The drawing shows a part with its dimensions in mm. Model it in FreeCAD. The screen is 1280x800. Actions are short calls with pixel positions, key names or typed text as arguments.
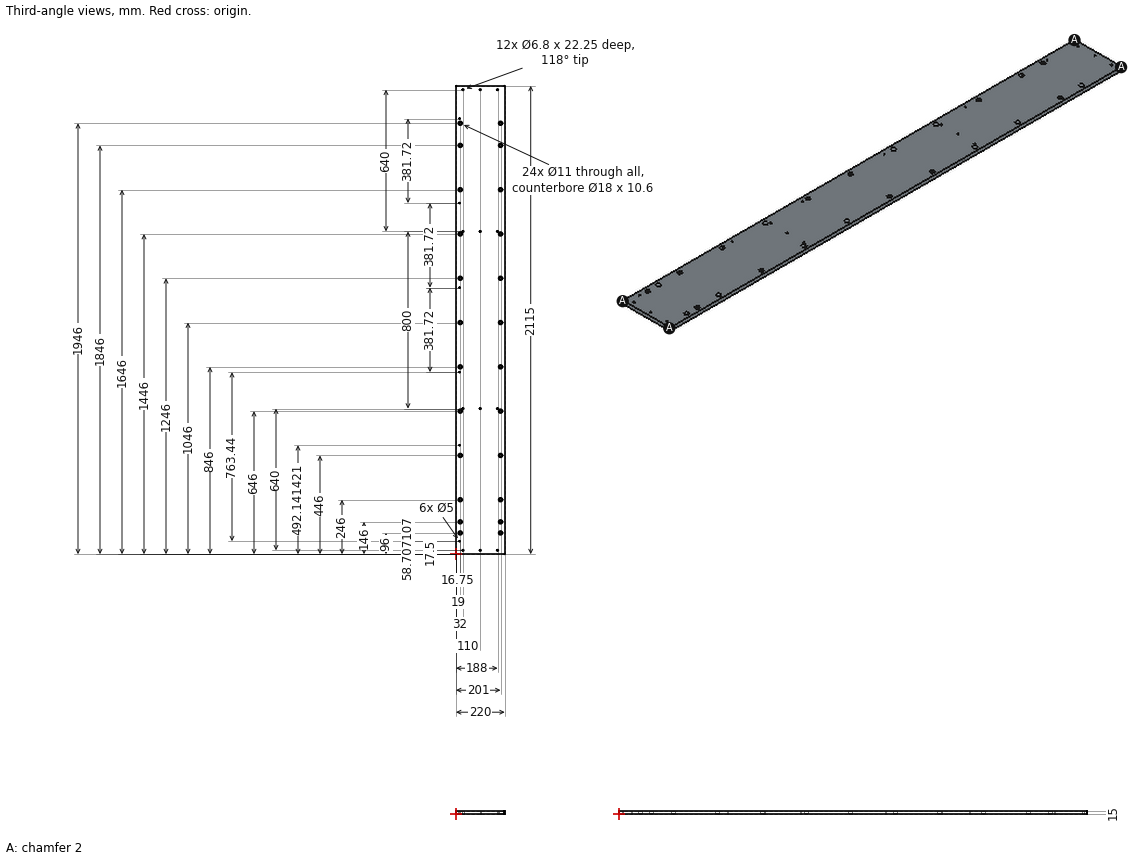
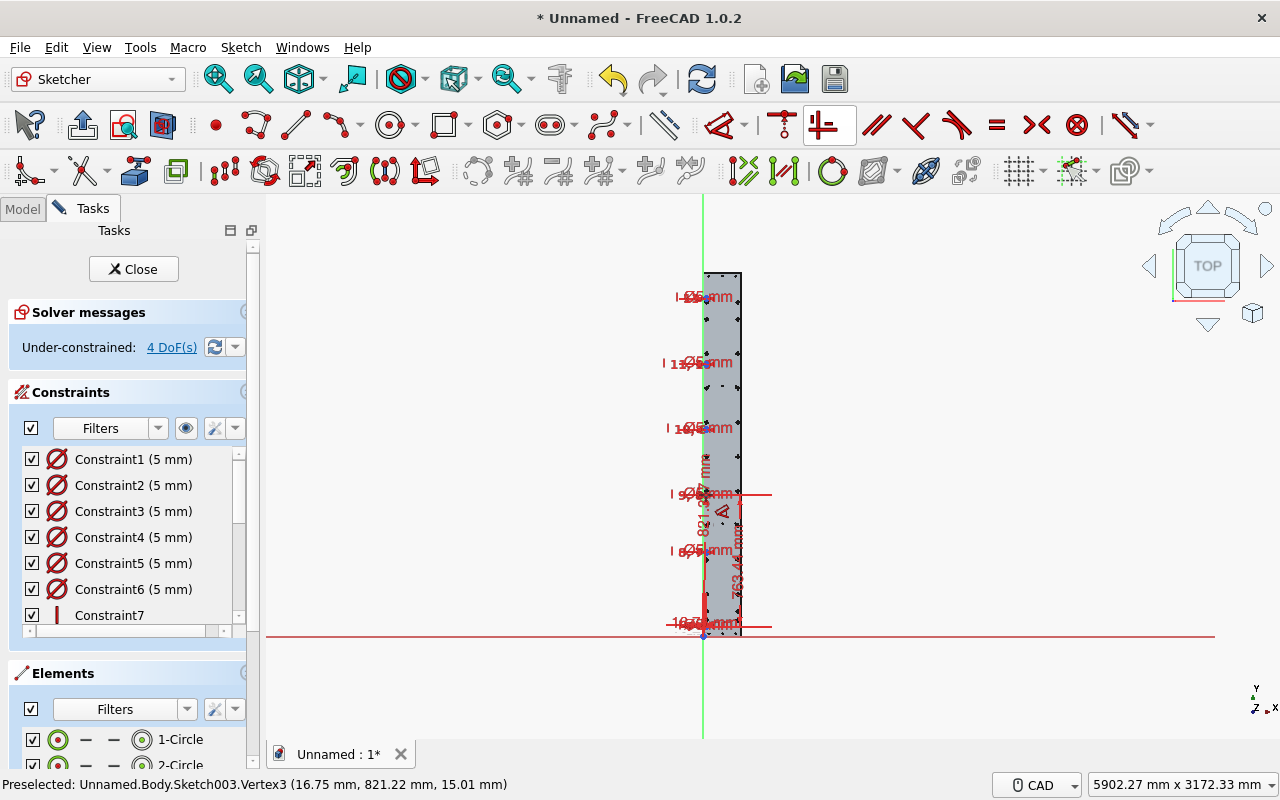
click(706, 430)
click(740, 463)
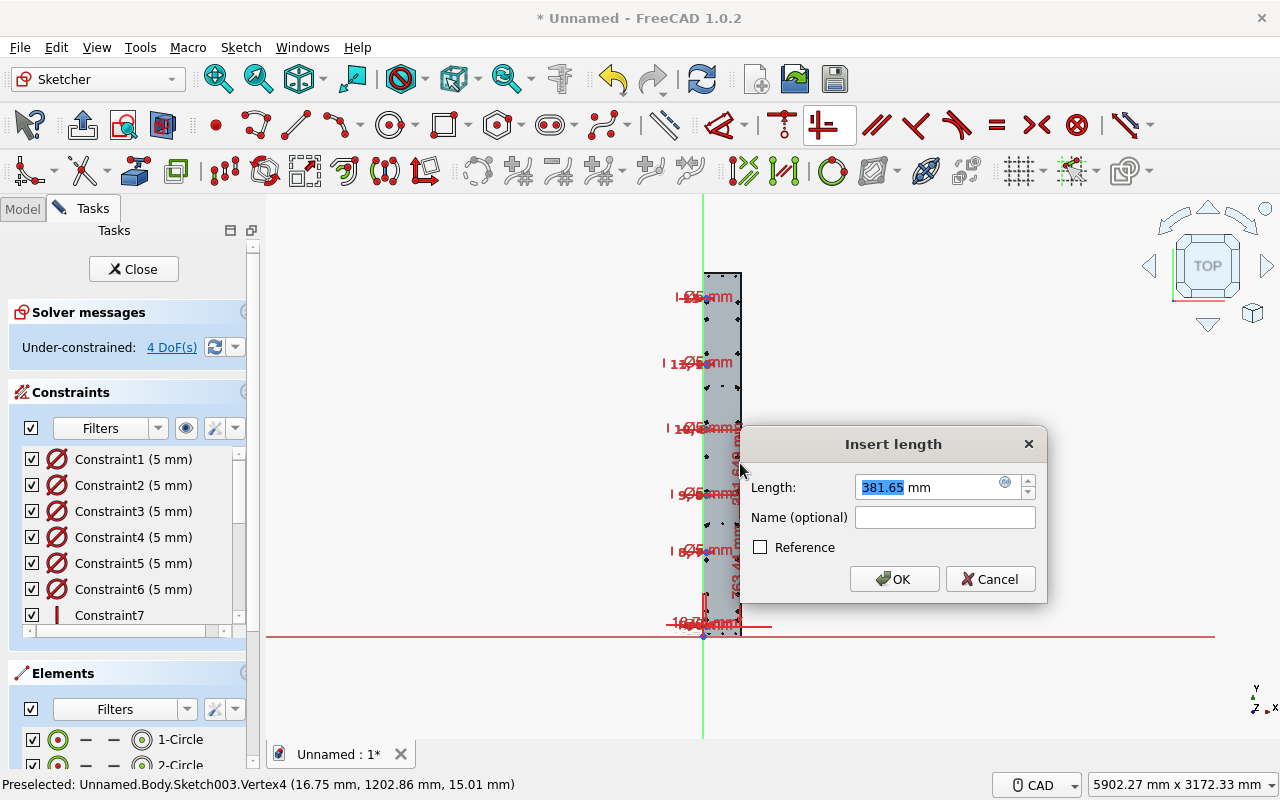
text(381.72)
key(Return)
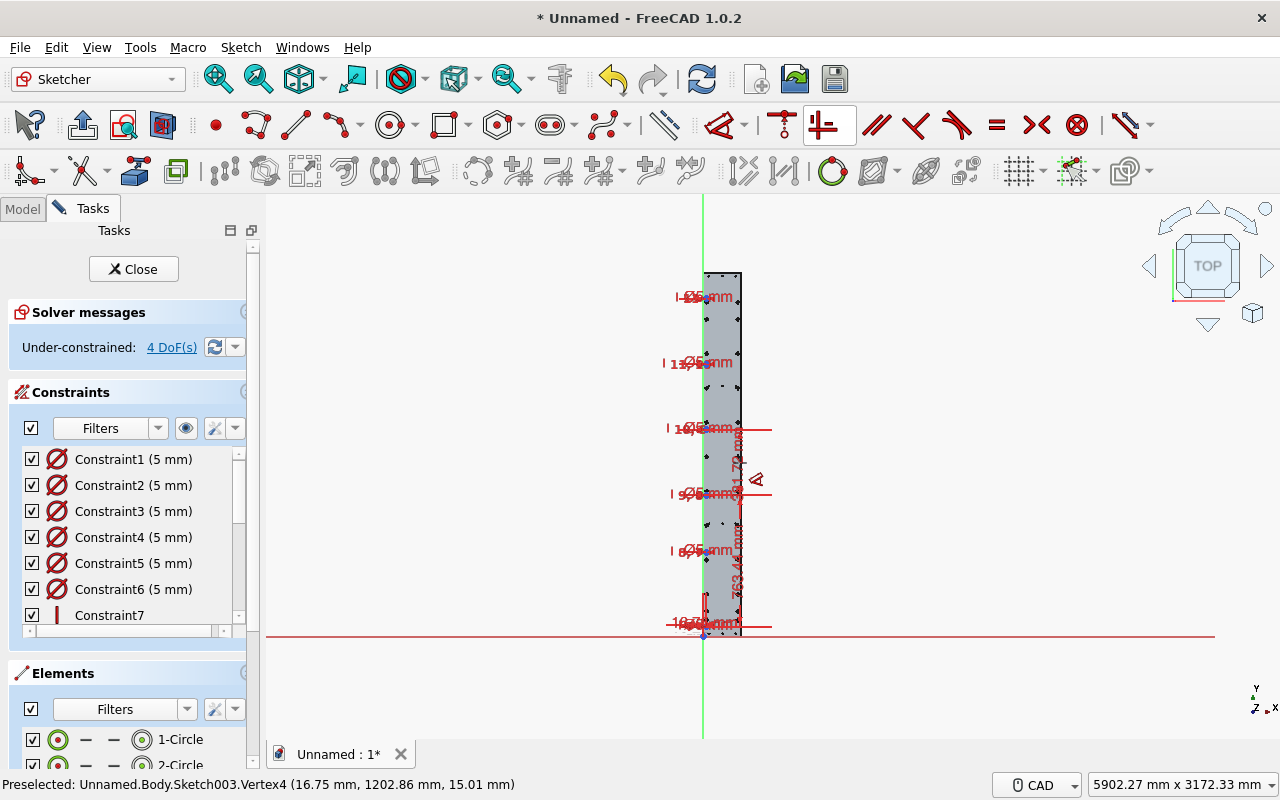
click(706, 430)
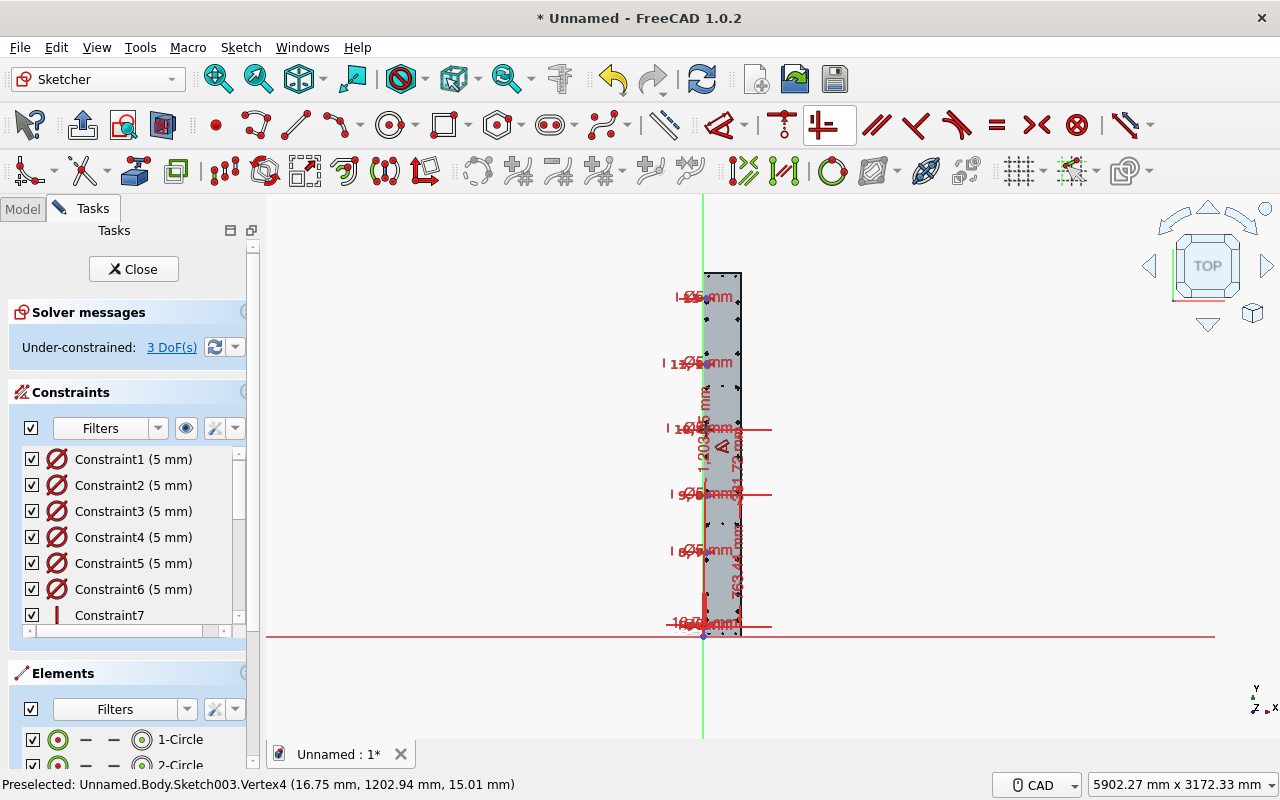
click(706, 364)
click(740, 397)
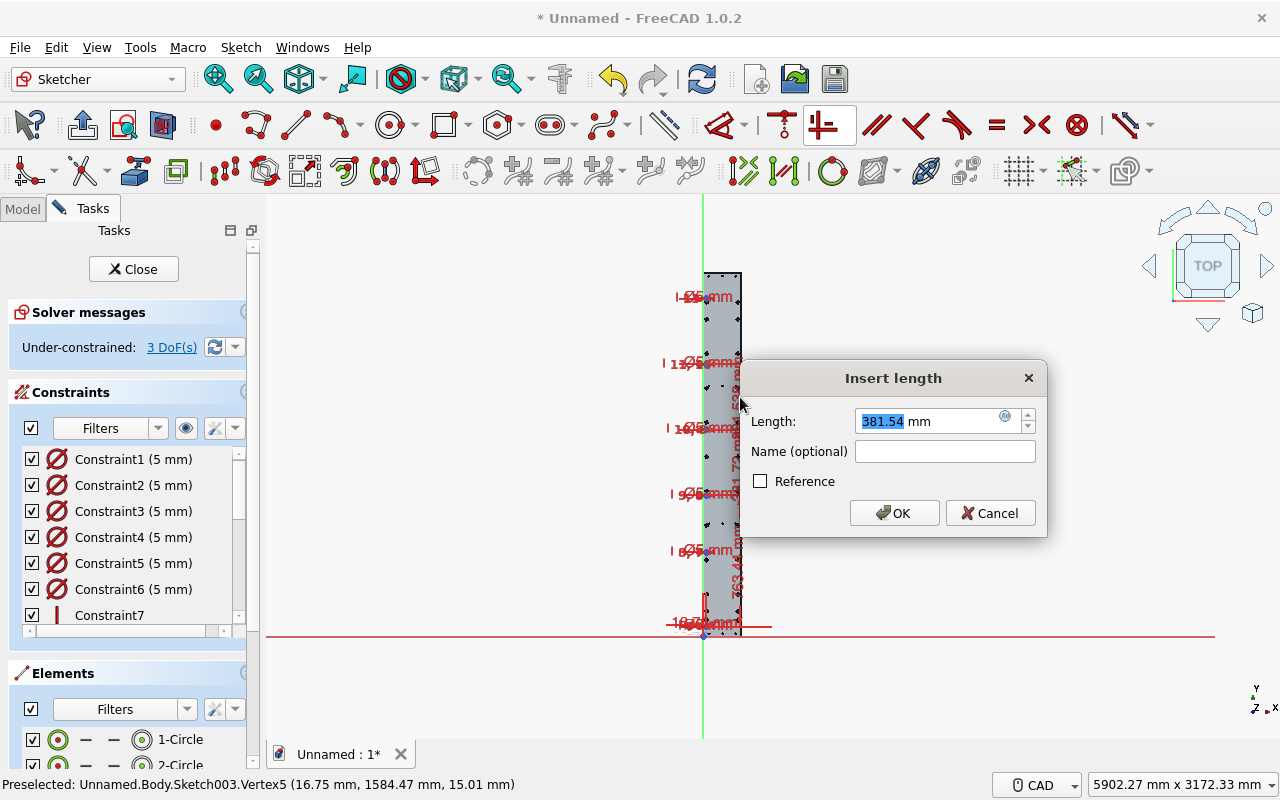
text(381.72)
key(Return)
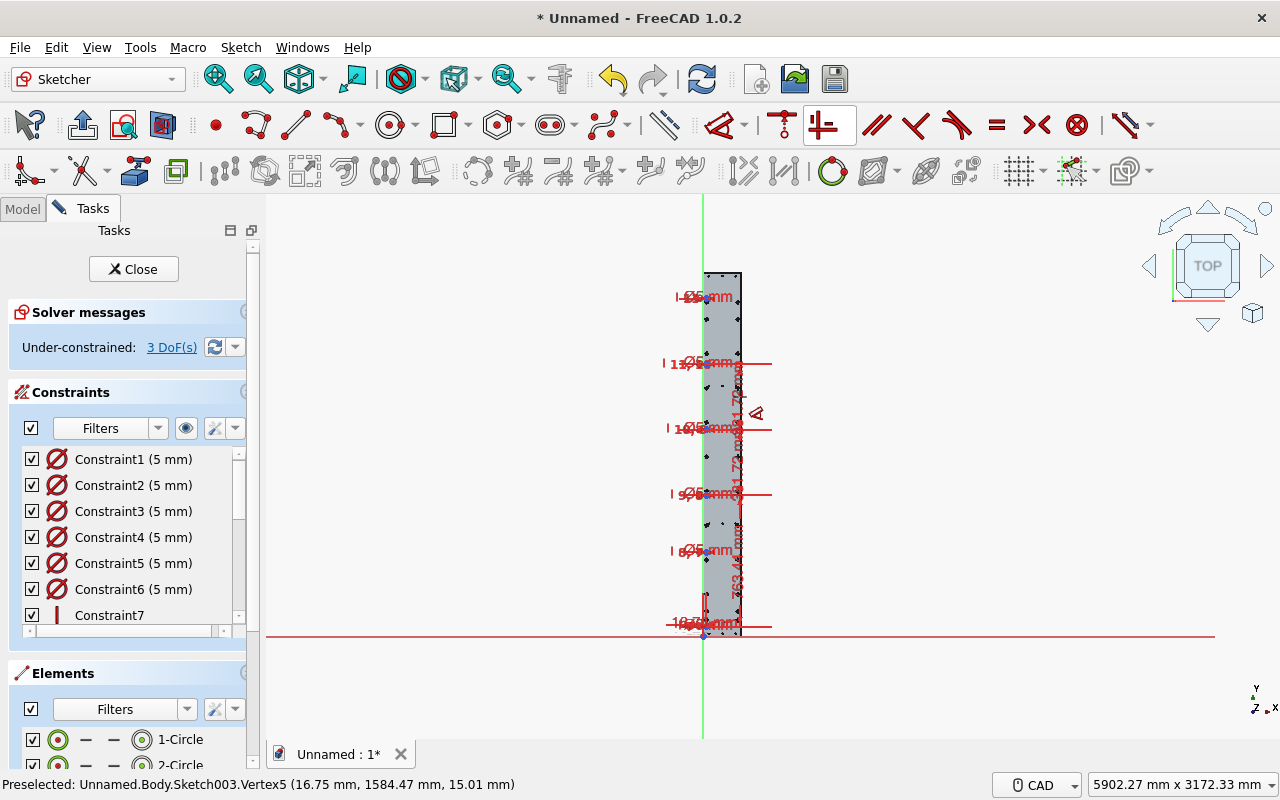
click(706, 364)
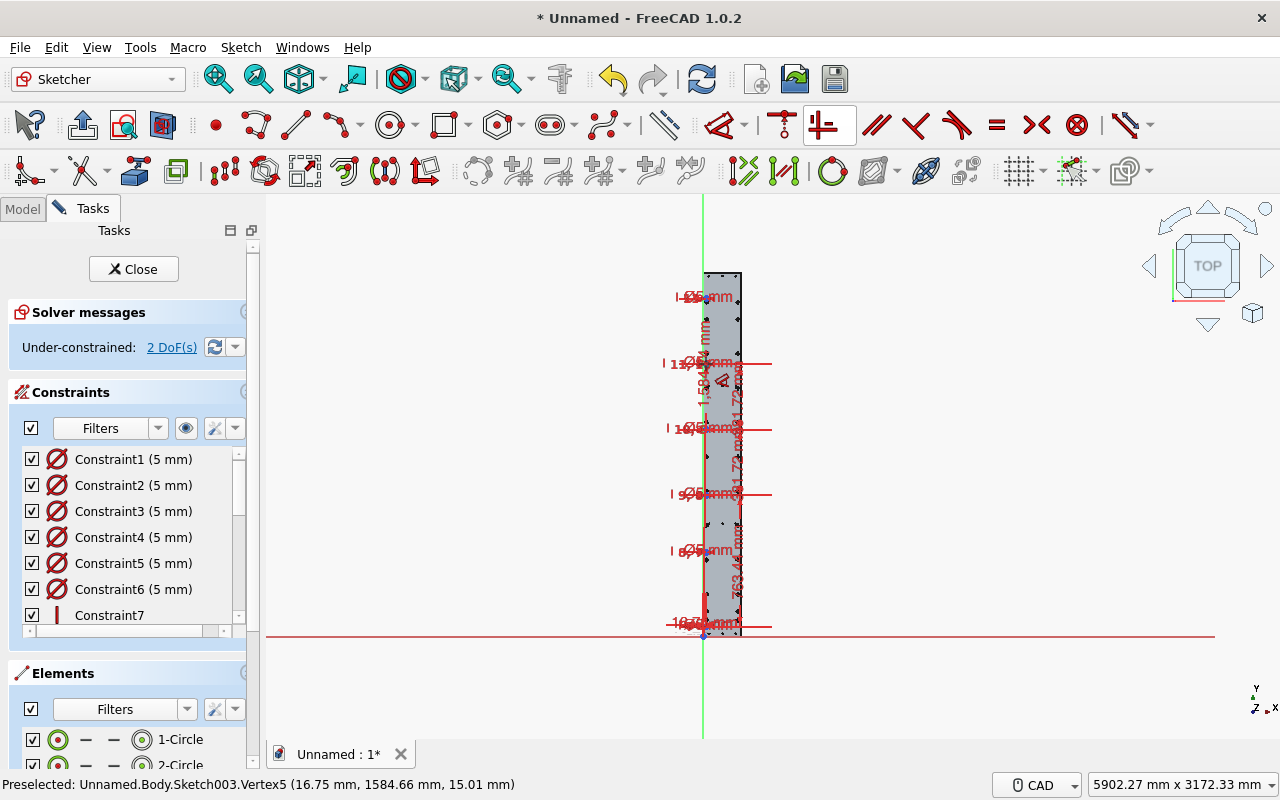
click(706, 299)
click(740, 332)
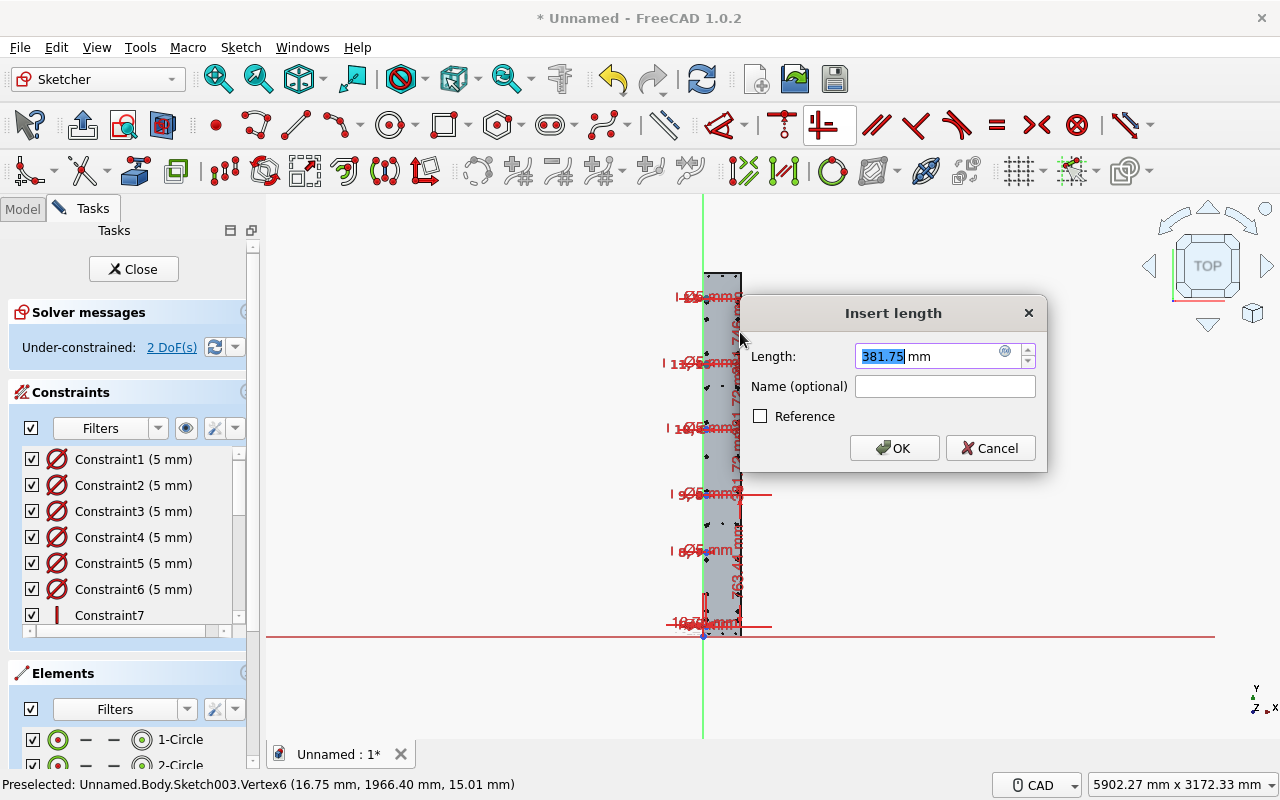
text(381.72)
key(Return)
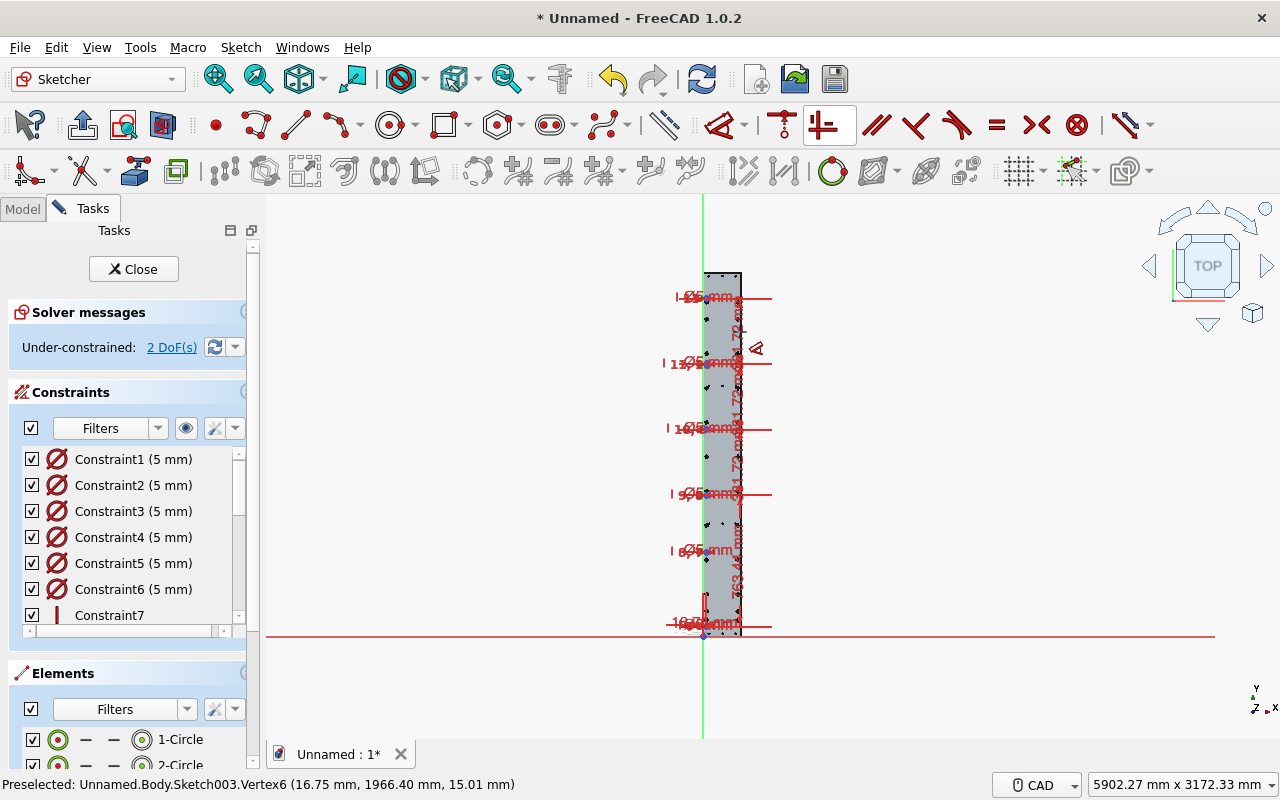
scroll(706, 627, up, 7)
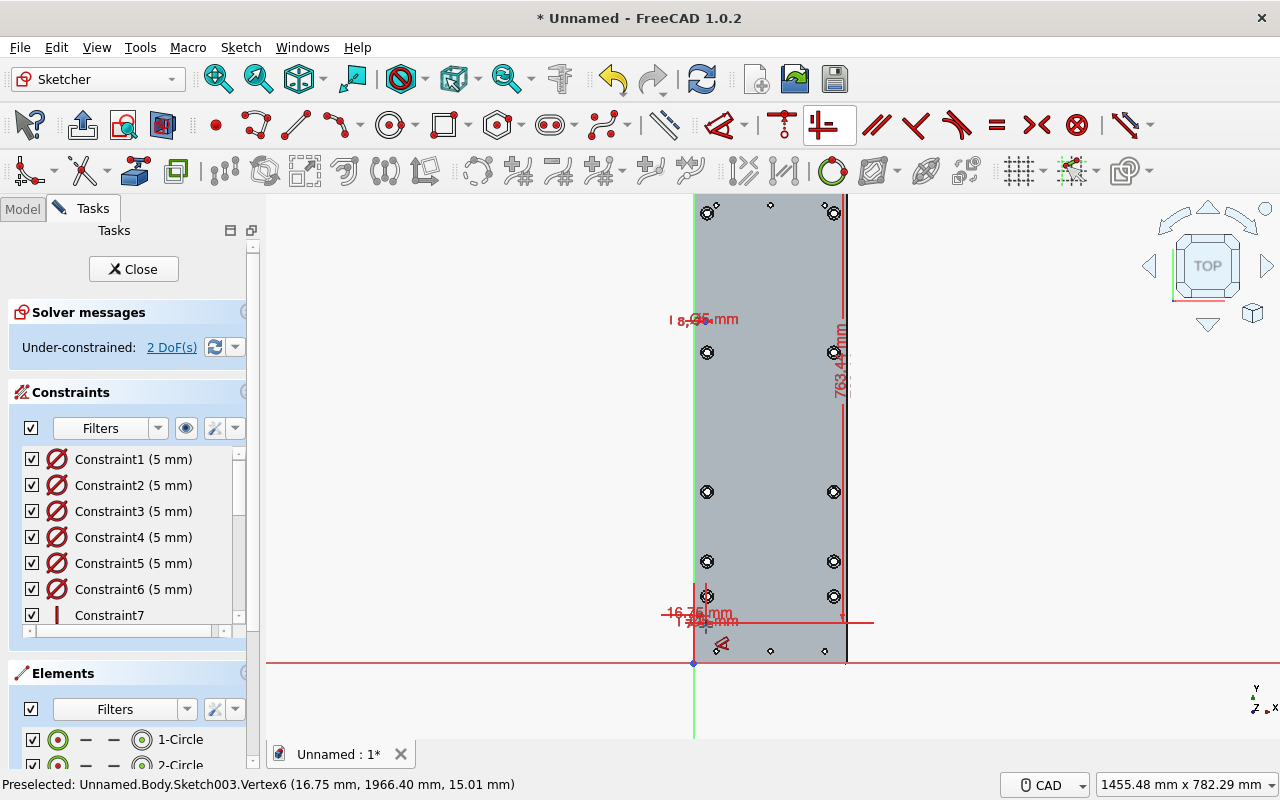
click(706, 623)
click(660, 643)